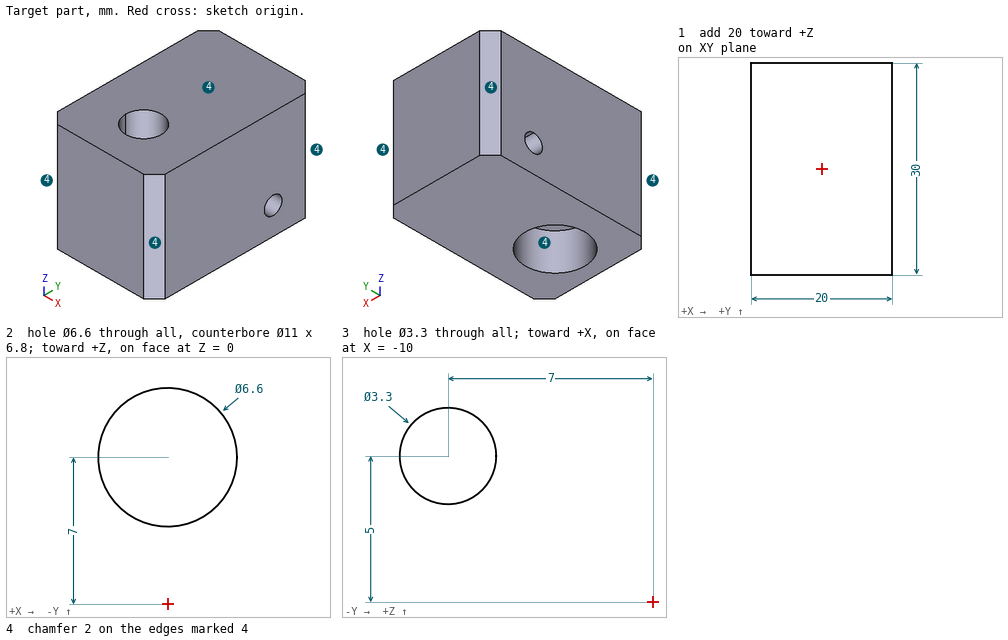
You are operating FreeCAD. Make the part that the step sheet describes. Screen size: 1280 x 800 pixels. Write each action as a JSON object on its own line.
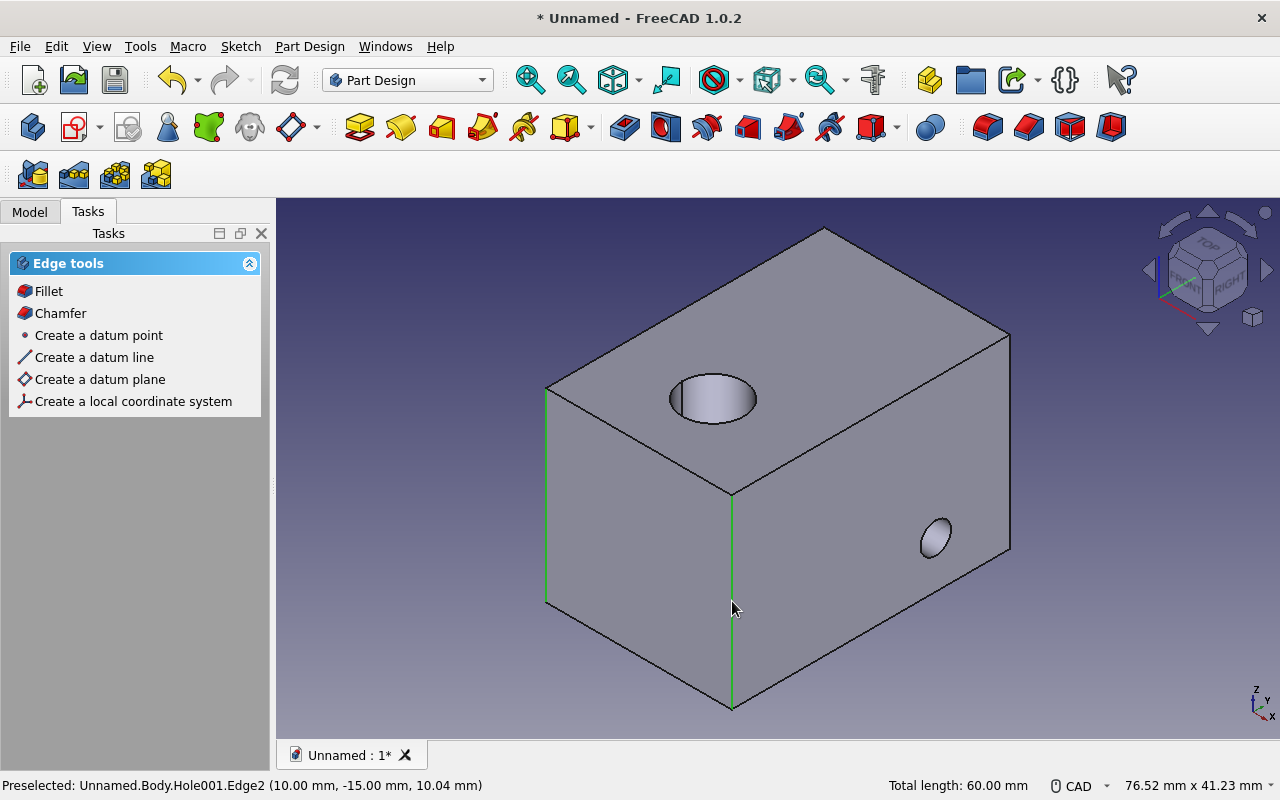
{"action": "key", "text": "2"}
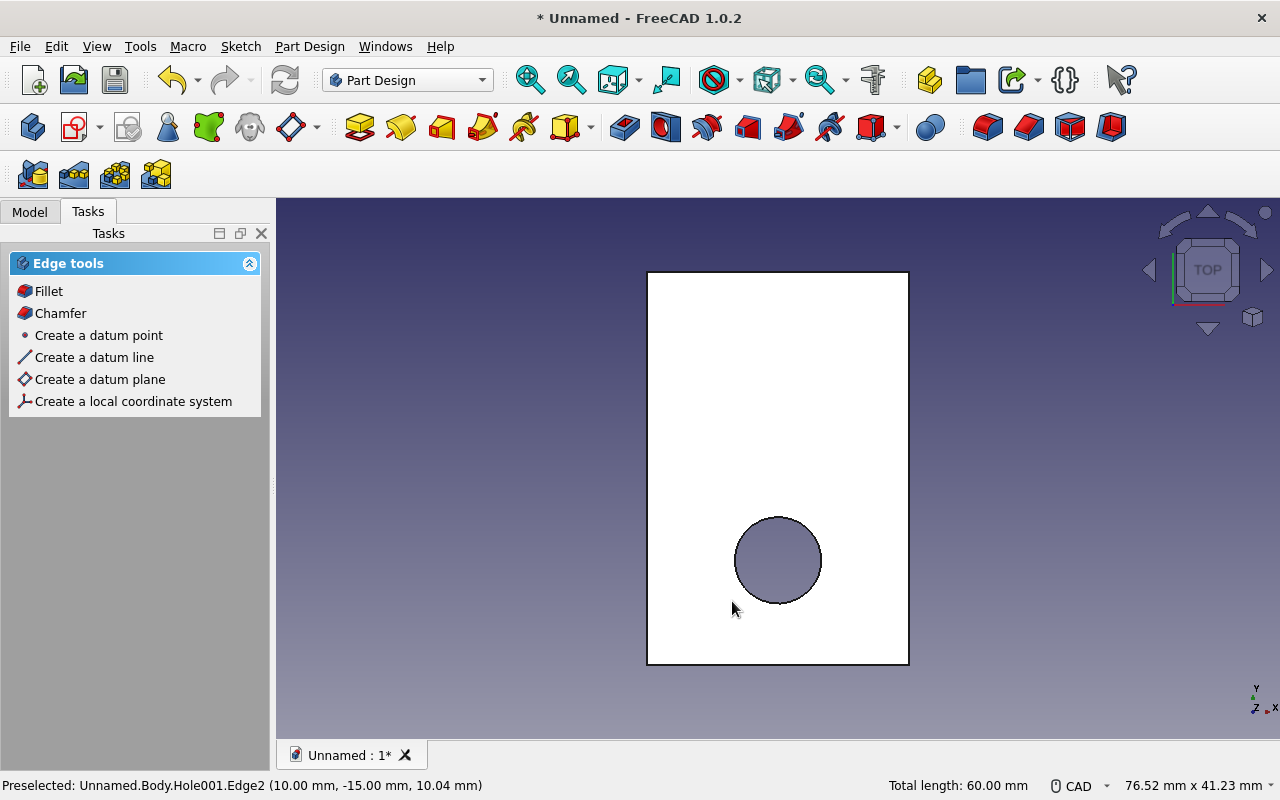
{"action": "key", "text": "1"}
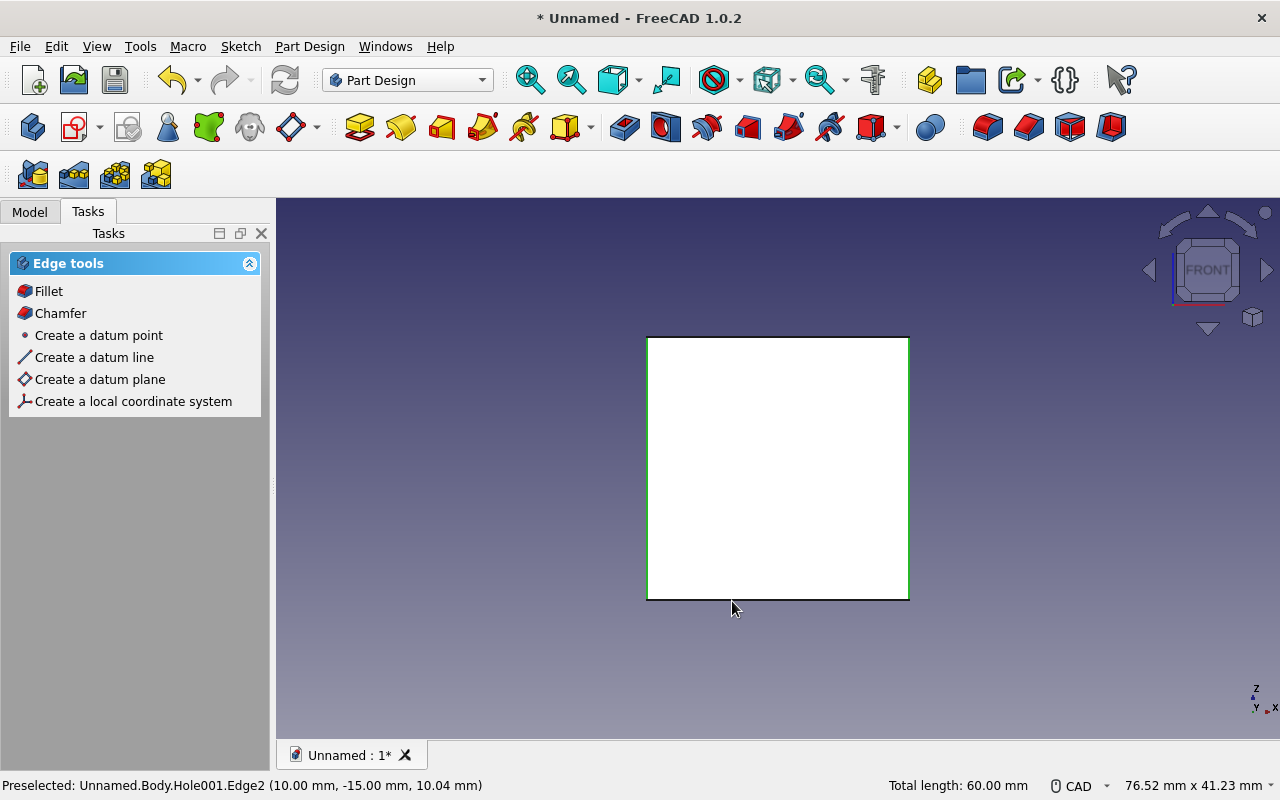
{"action": "key", "text": "3"}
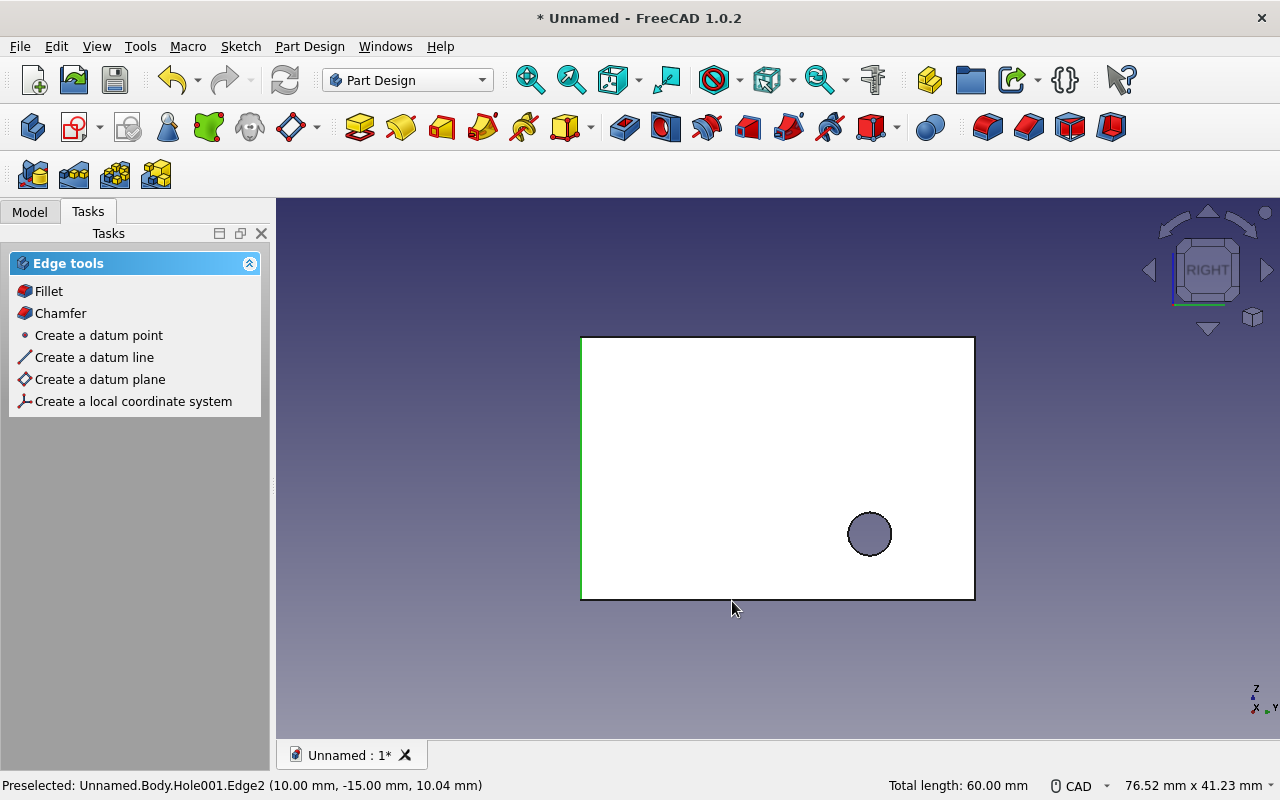
{"action": "left_click", "coordinate": [975, 468], "text": "ctrl"}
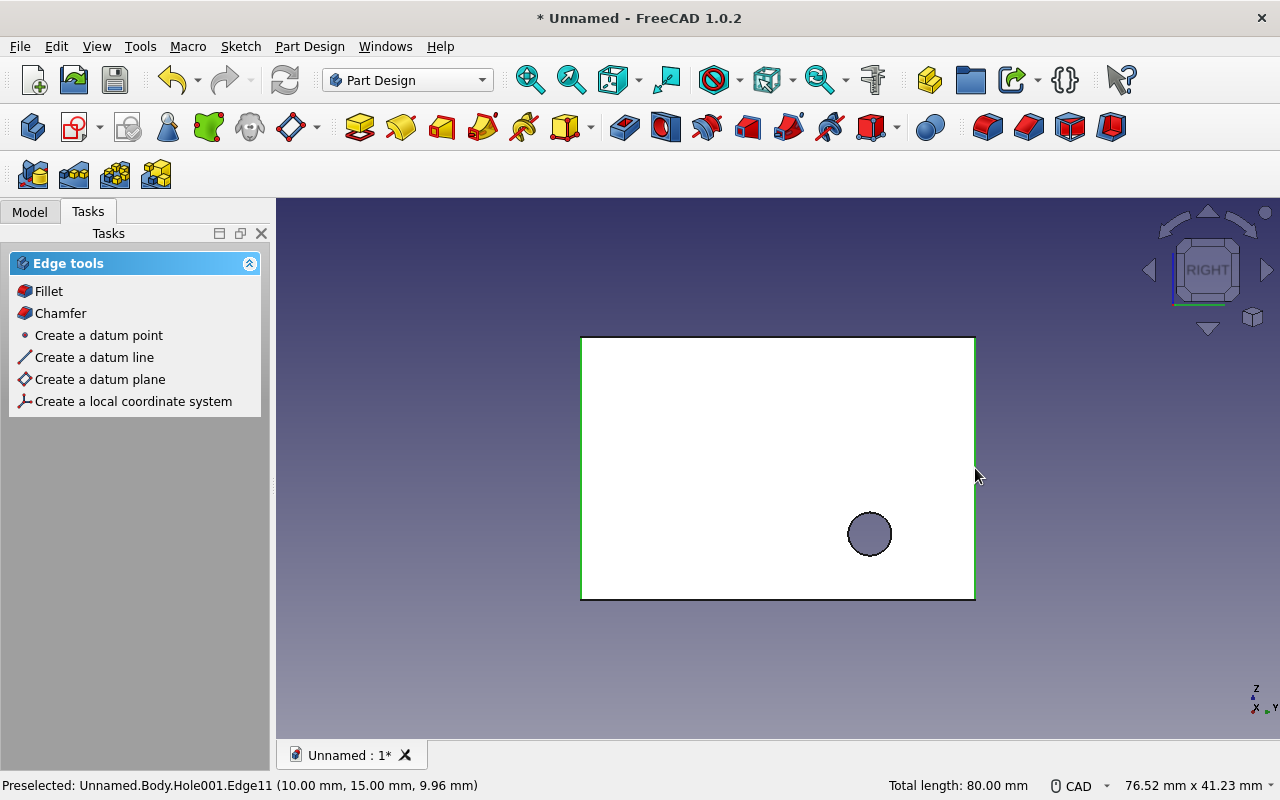
{"action": "left_click", "coordinate": [1029, 128]}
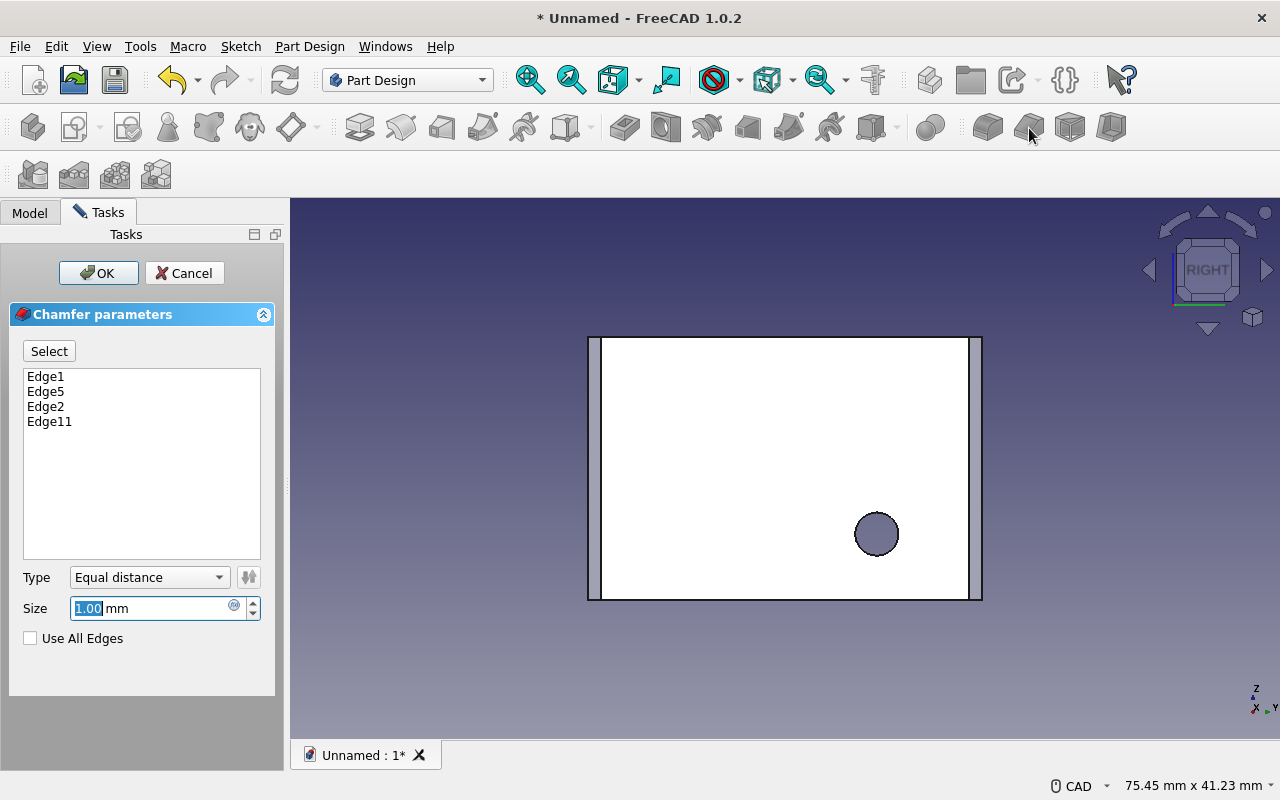
{"action": "type", "text": "2"}
{"action": "key", "text": "Tab"}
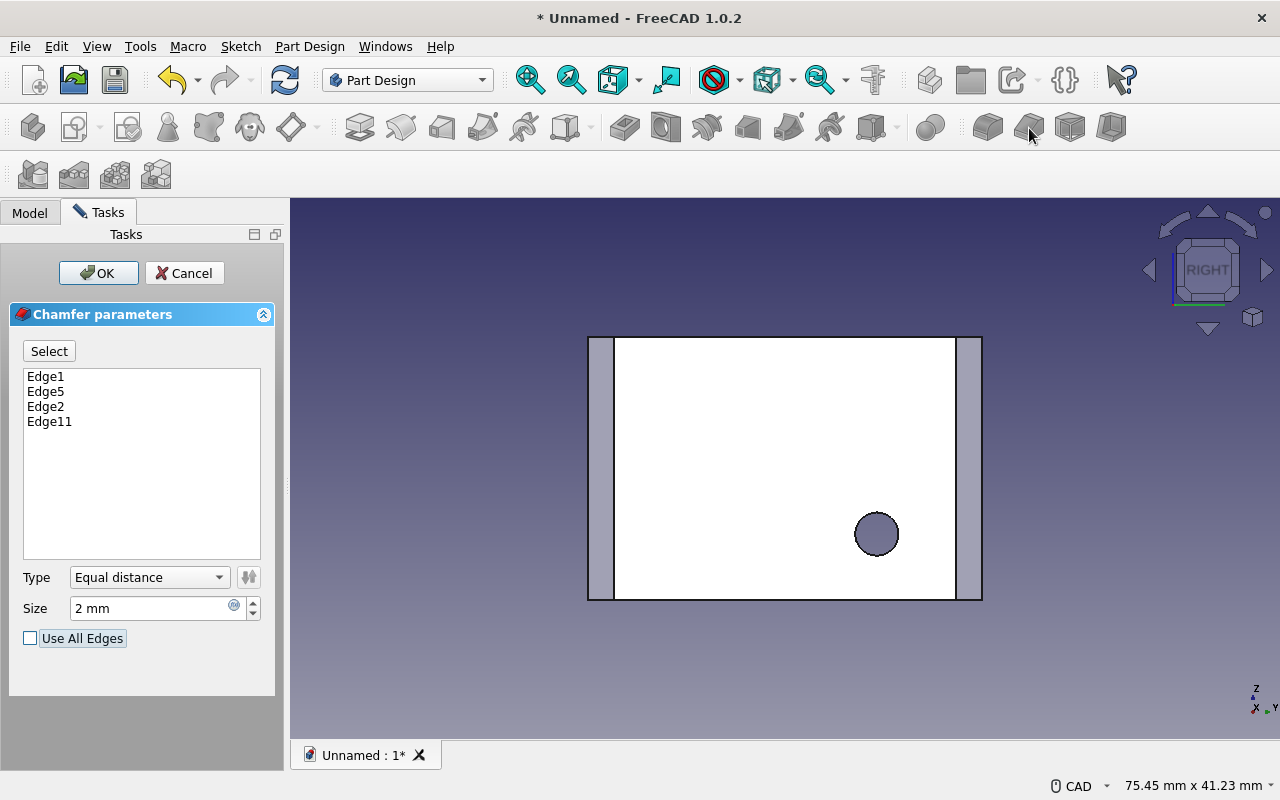
{"action": "left_click", "coordinate": [99, 273]}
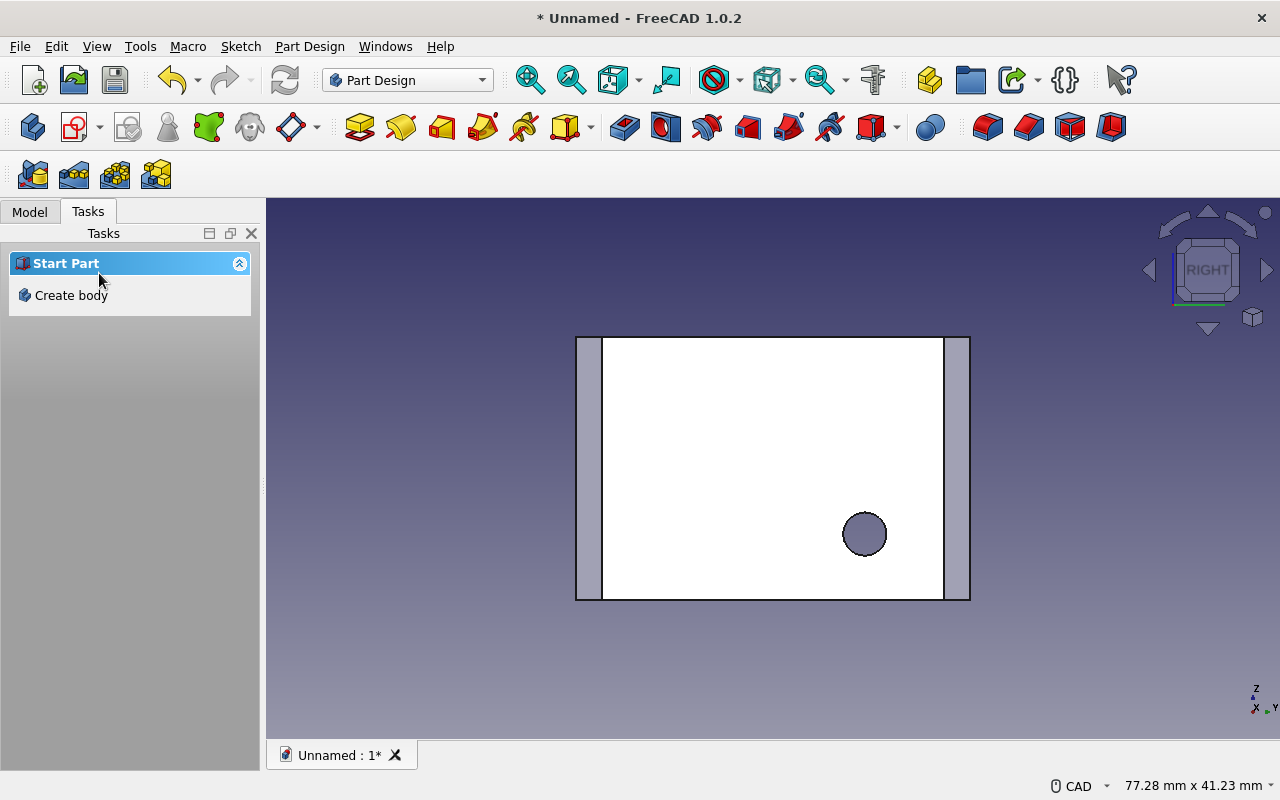
{"action": "key", "text": "0"}